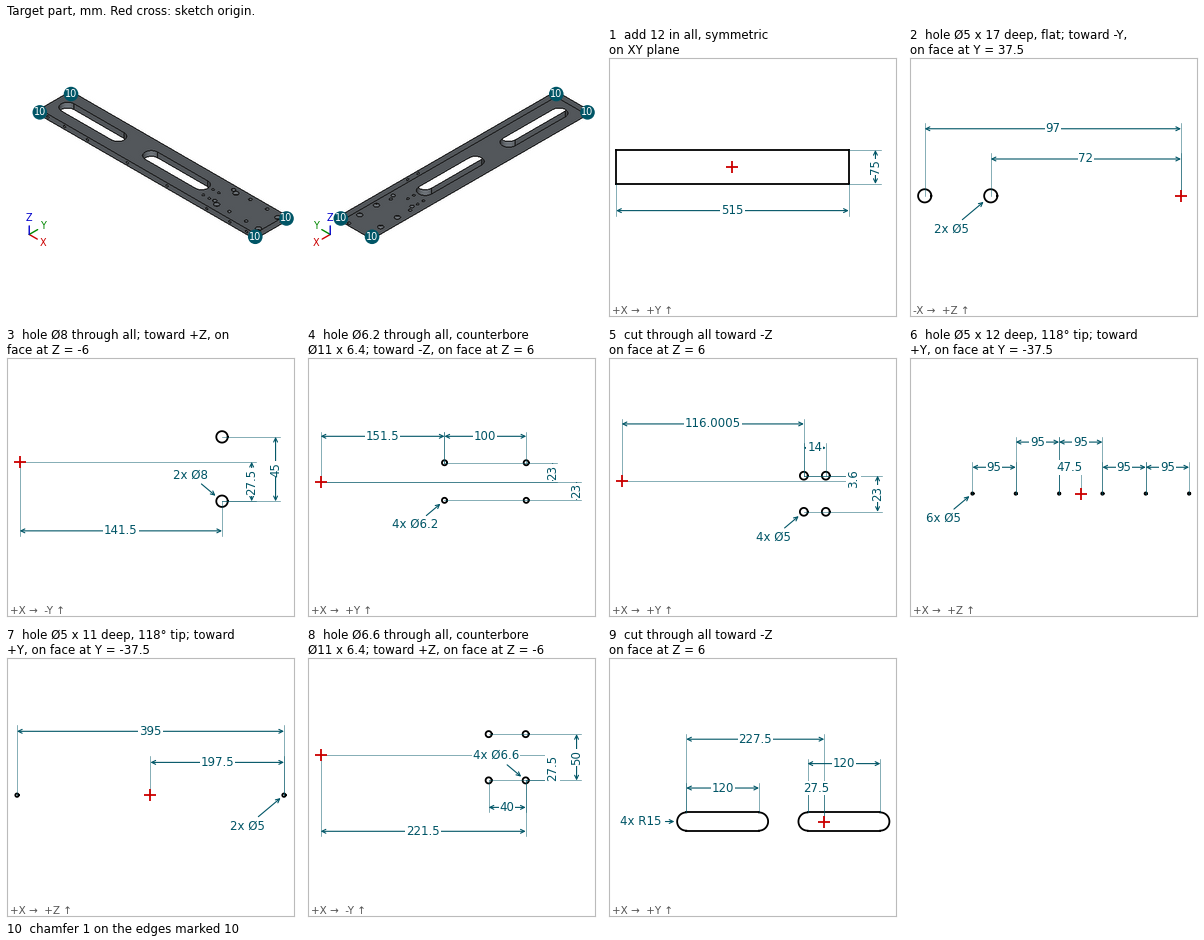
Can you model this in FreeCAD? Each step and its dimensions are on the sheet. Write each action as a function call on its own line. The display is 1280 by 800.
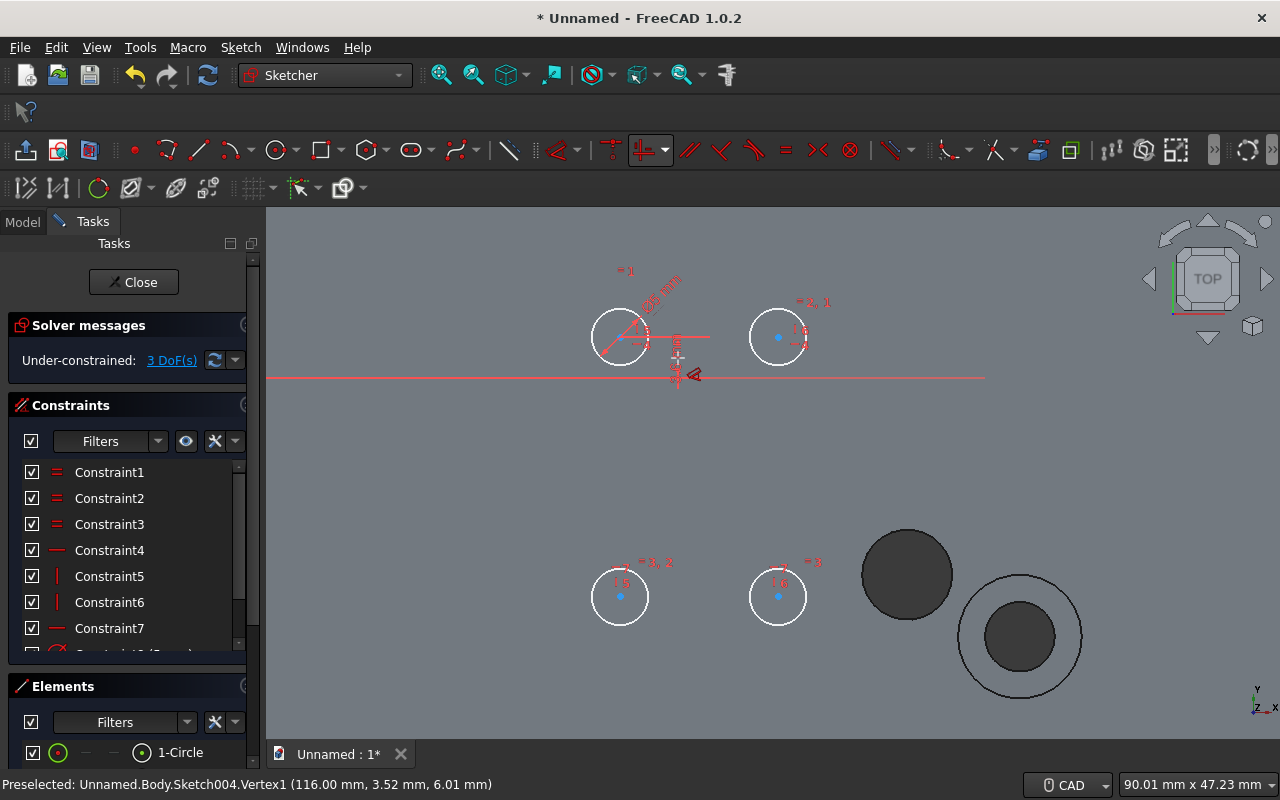
click(620, 337)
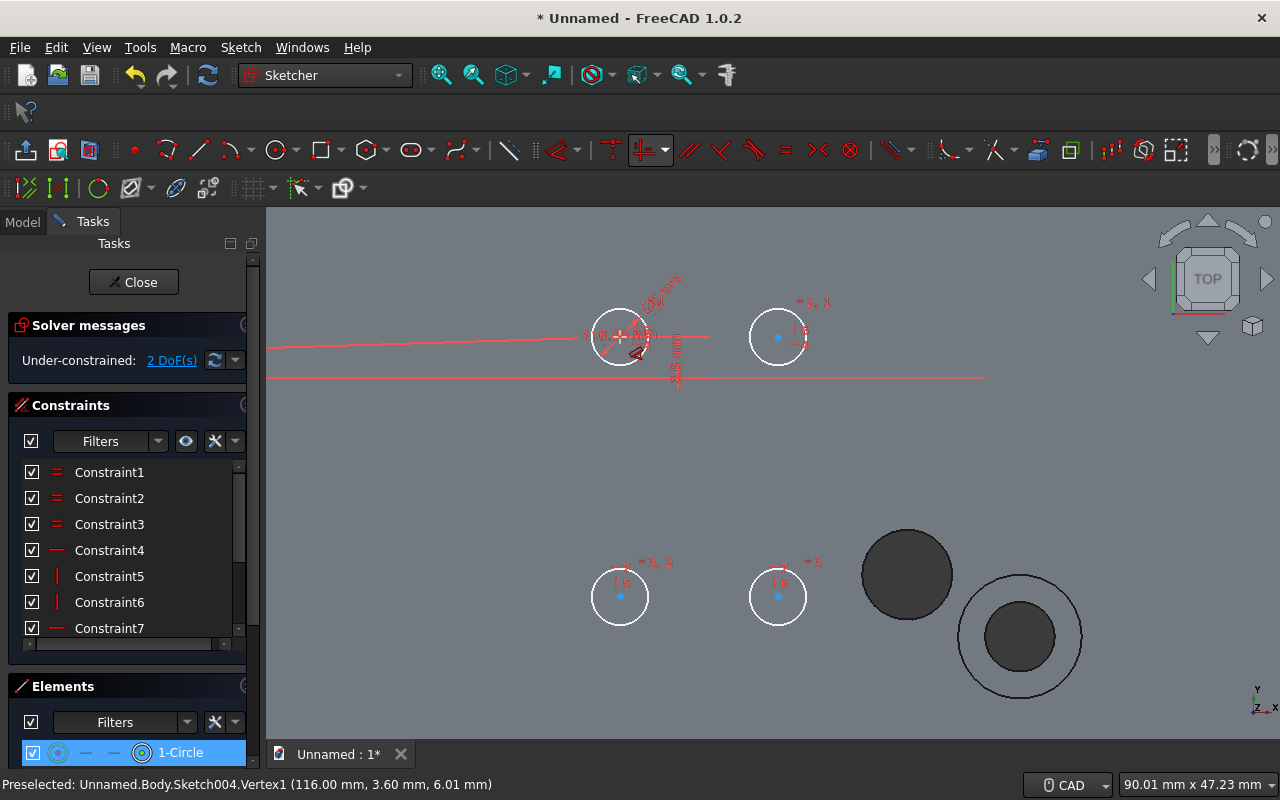
click(778, 337)
click(735, 303)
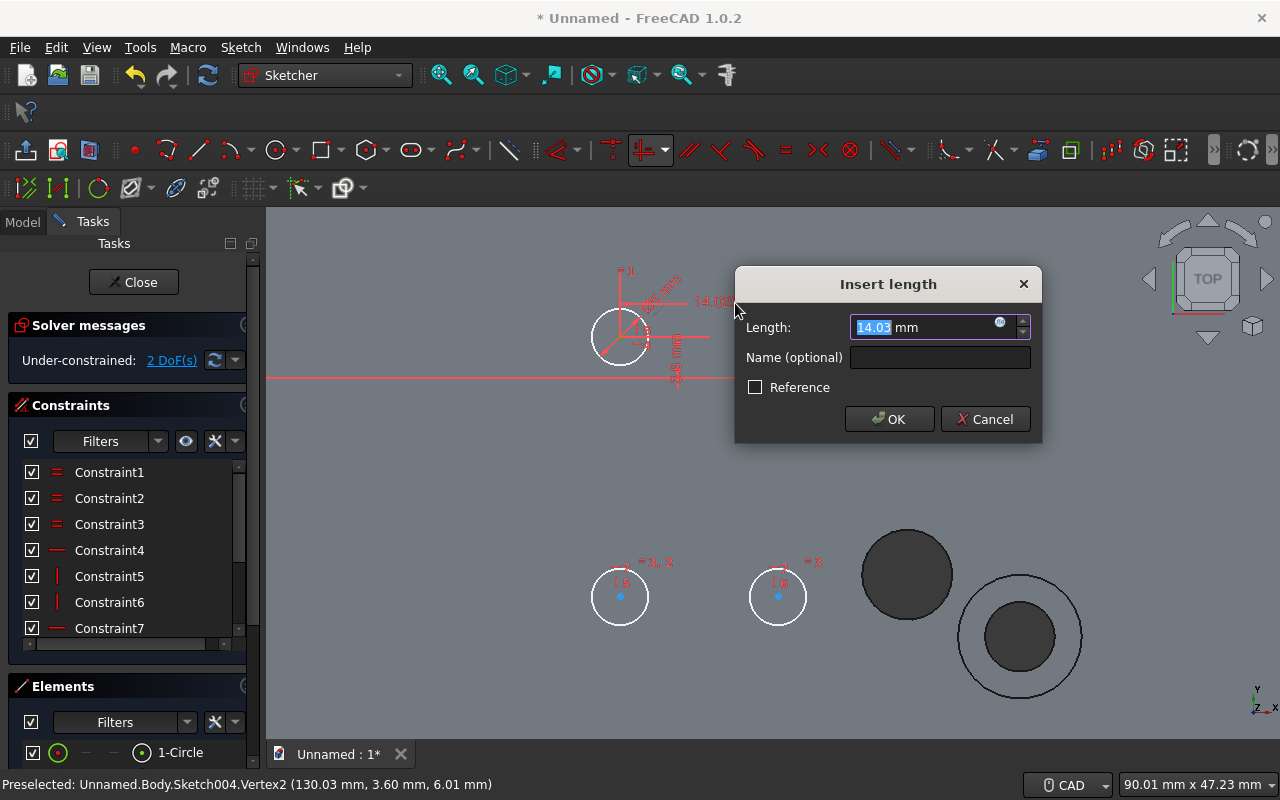
text(14)
key(Return)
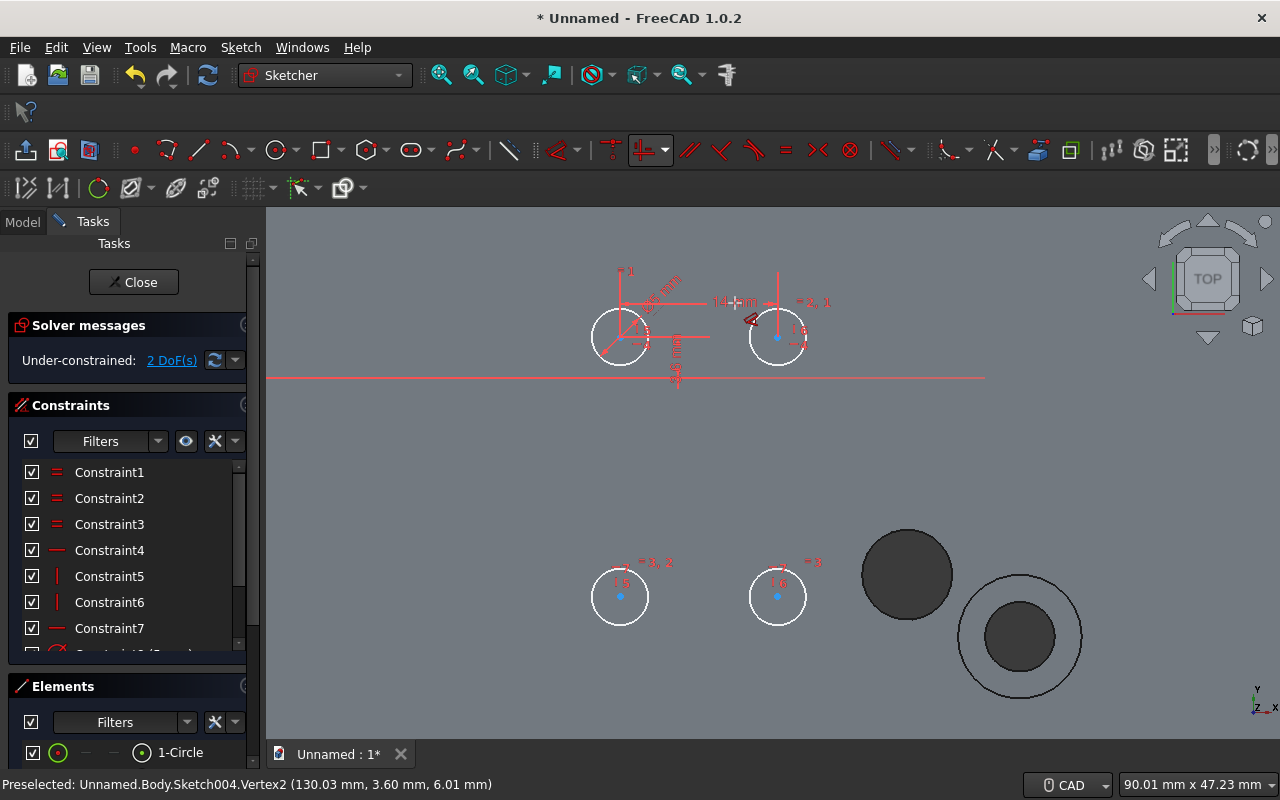
click(620, 337)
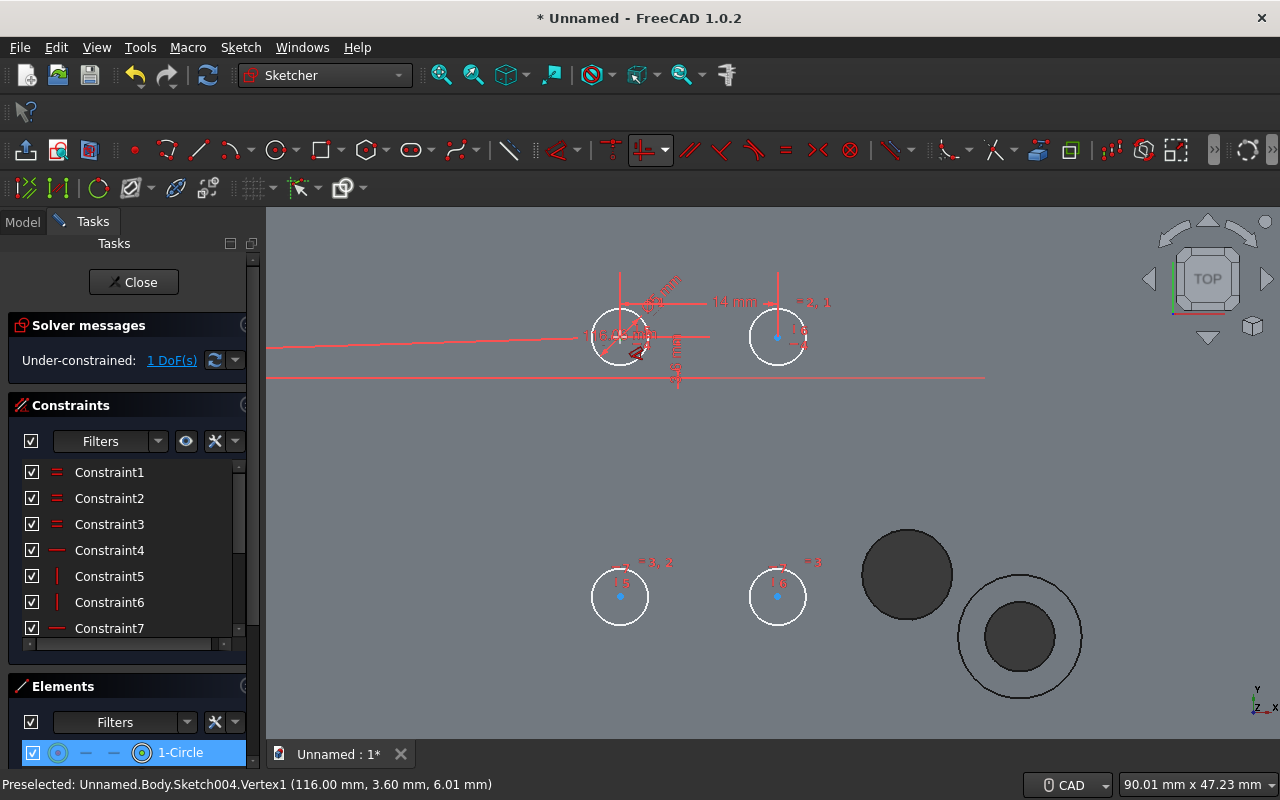
click(620, 597)
click(586, 467)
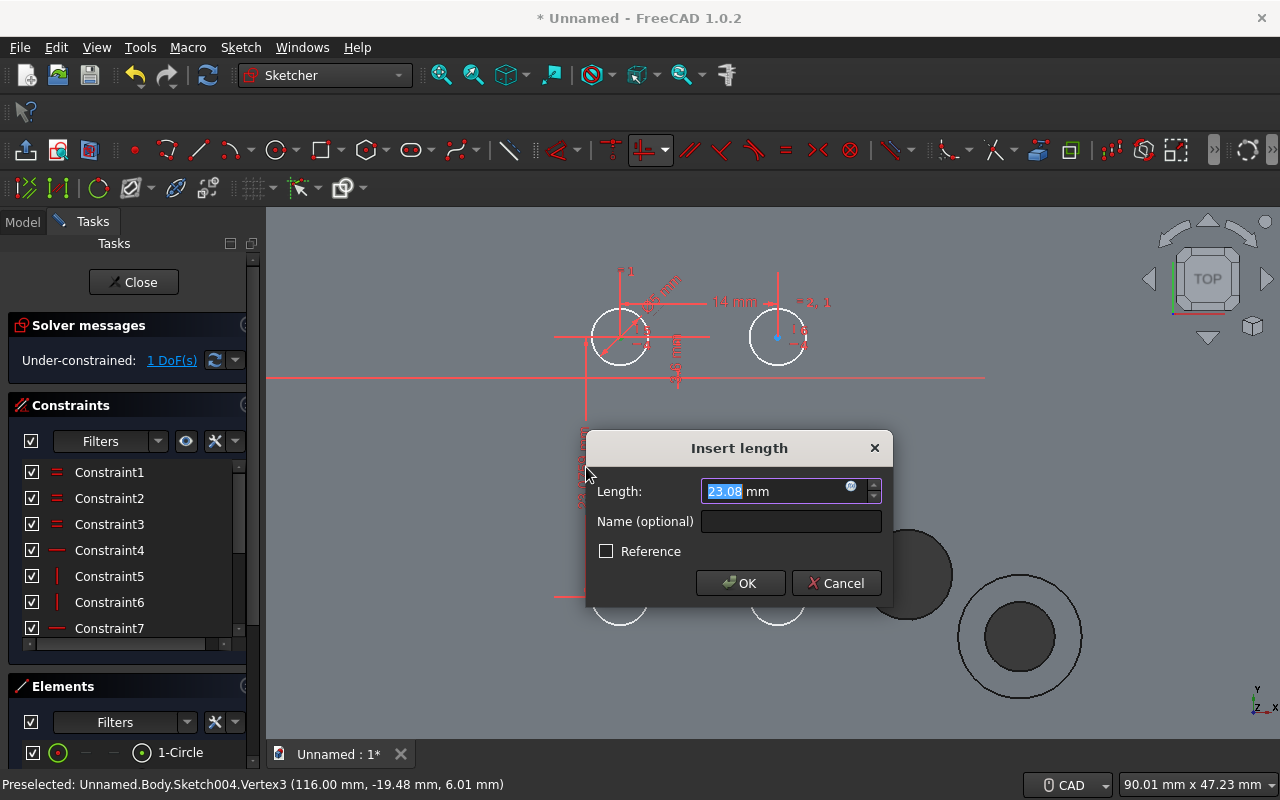
text(23)
key(Return)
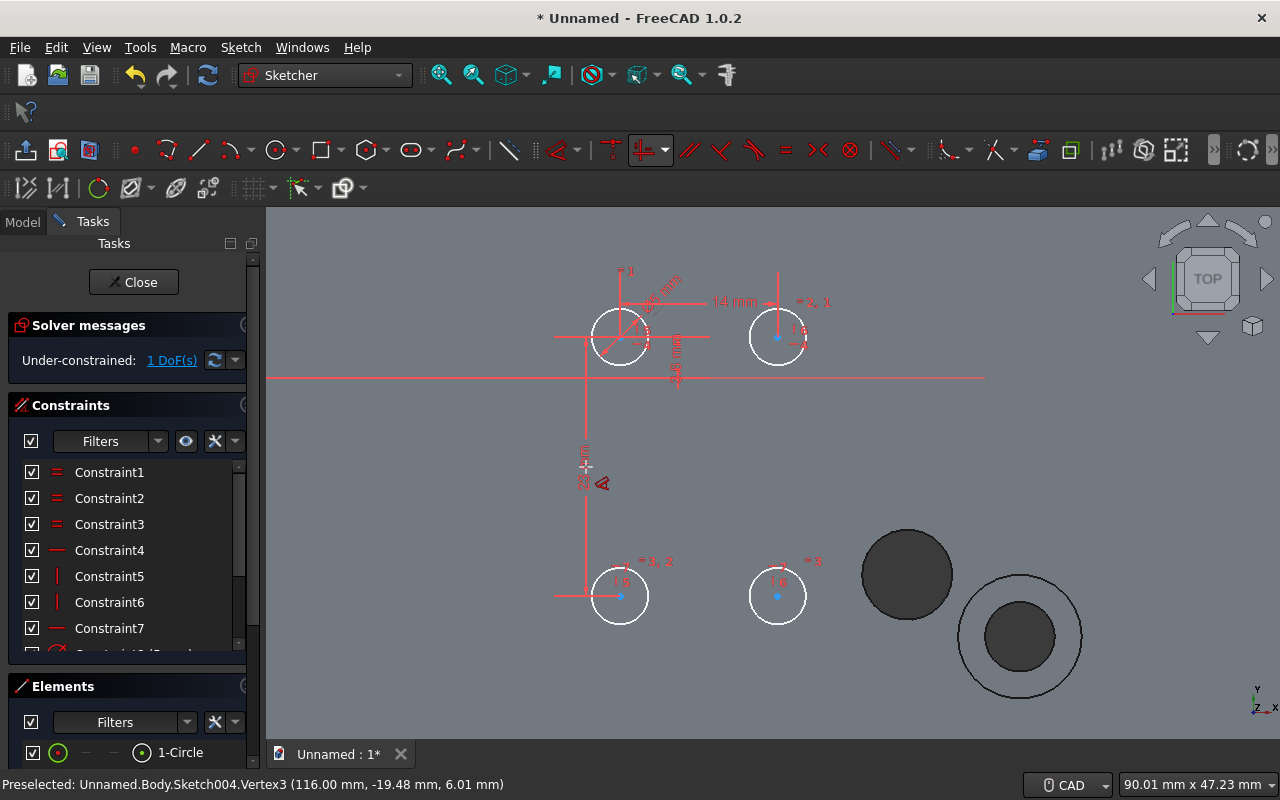
click(620, 337)
click(457, 303)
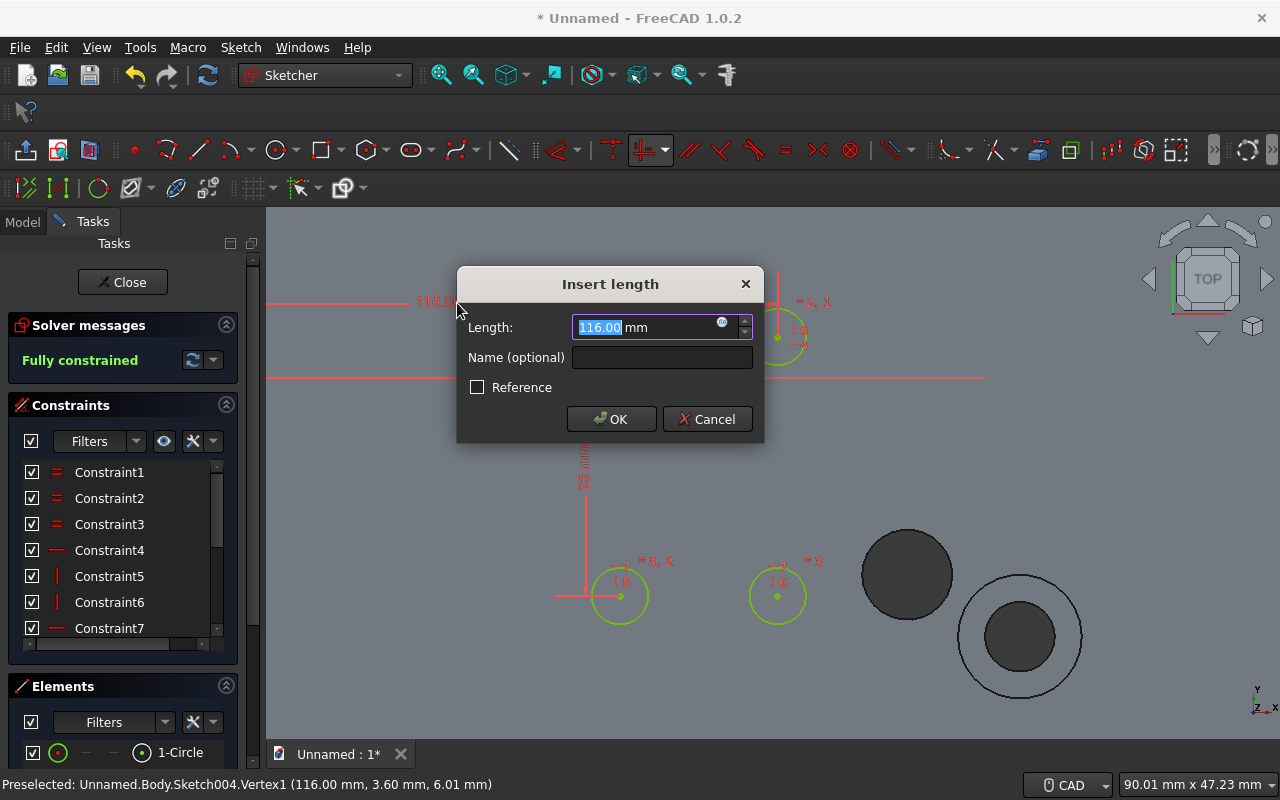
text(116.0005)
key(Return)
key(Escape)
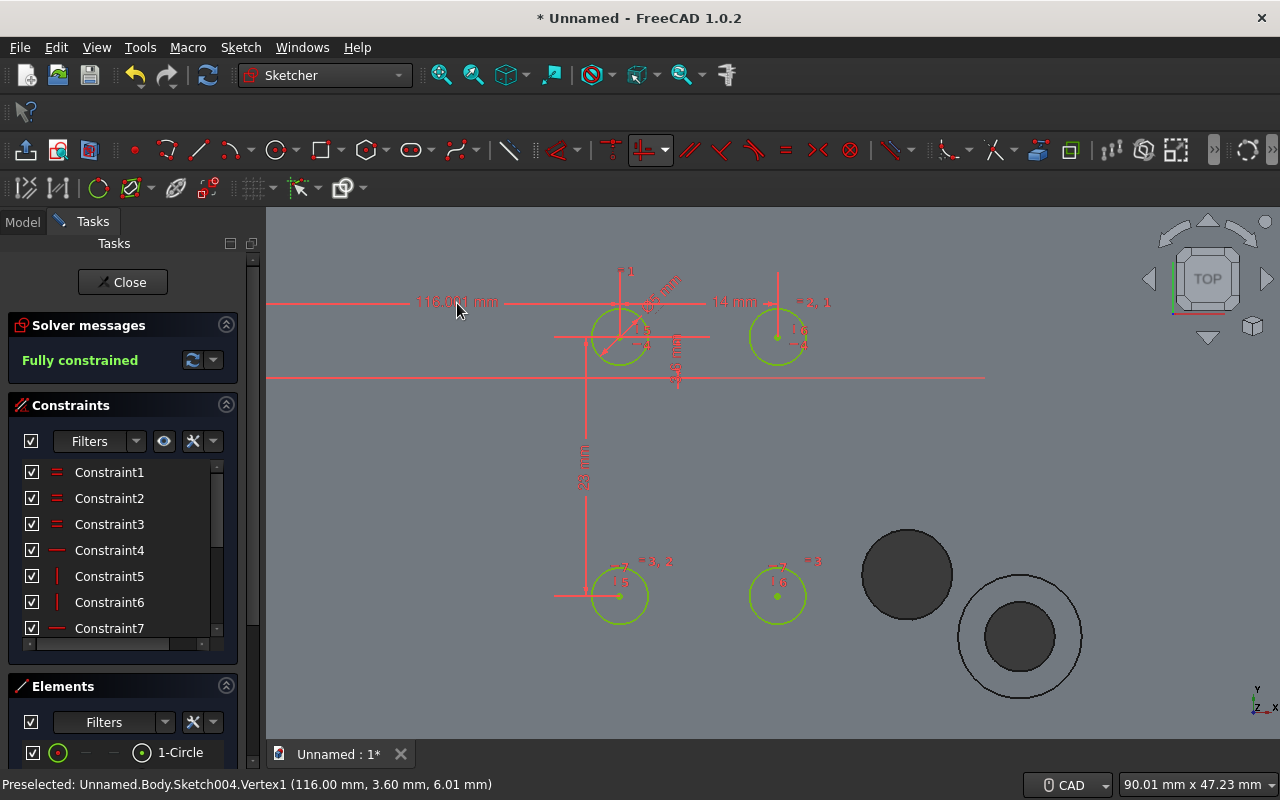
click(123, 282)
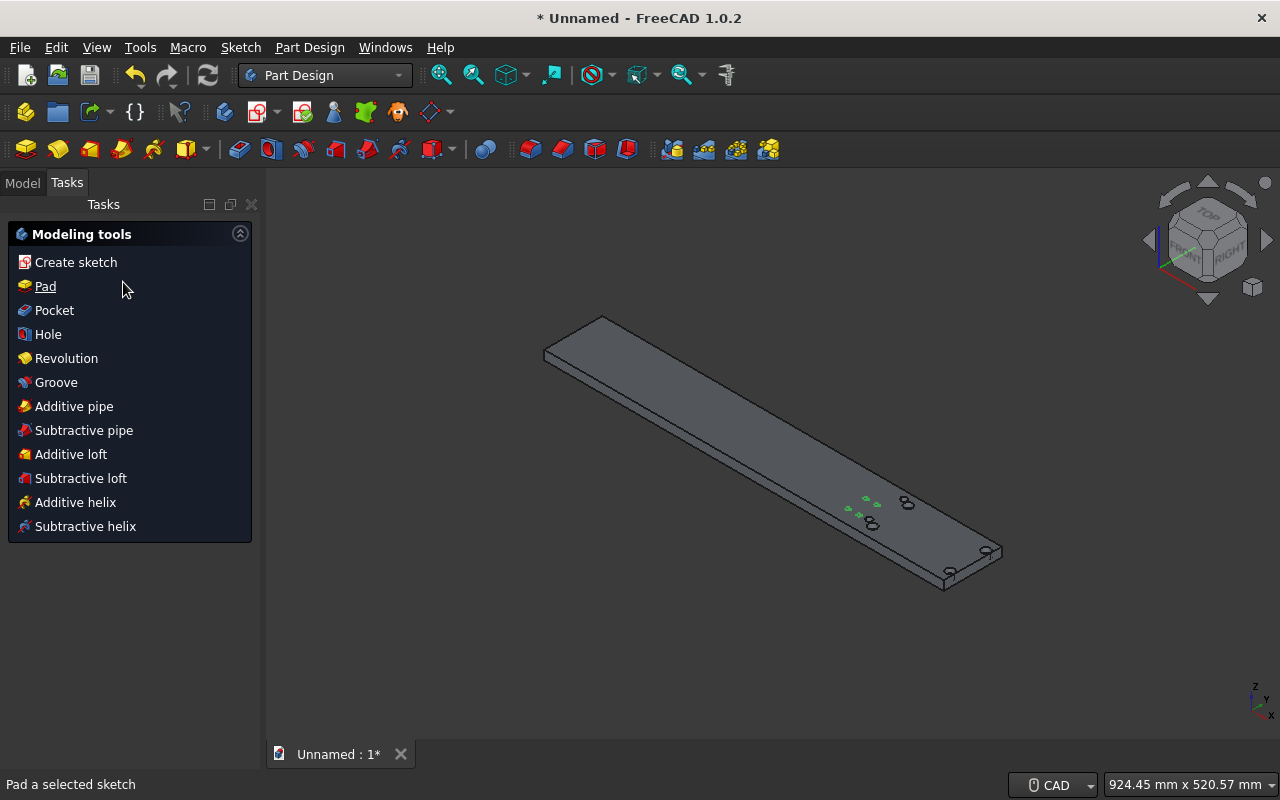
click(240, 150)